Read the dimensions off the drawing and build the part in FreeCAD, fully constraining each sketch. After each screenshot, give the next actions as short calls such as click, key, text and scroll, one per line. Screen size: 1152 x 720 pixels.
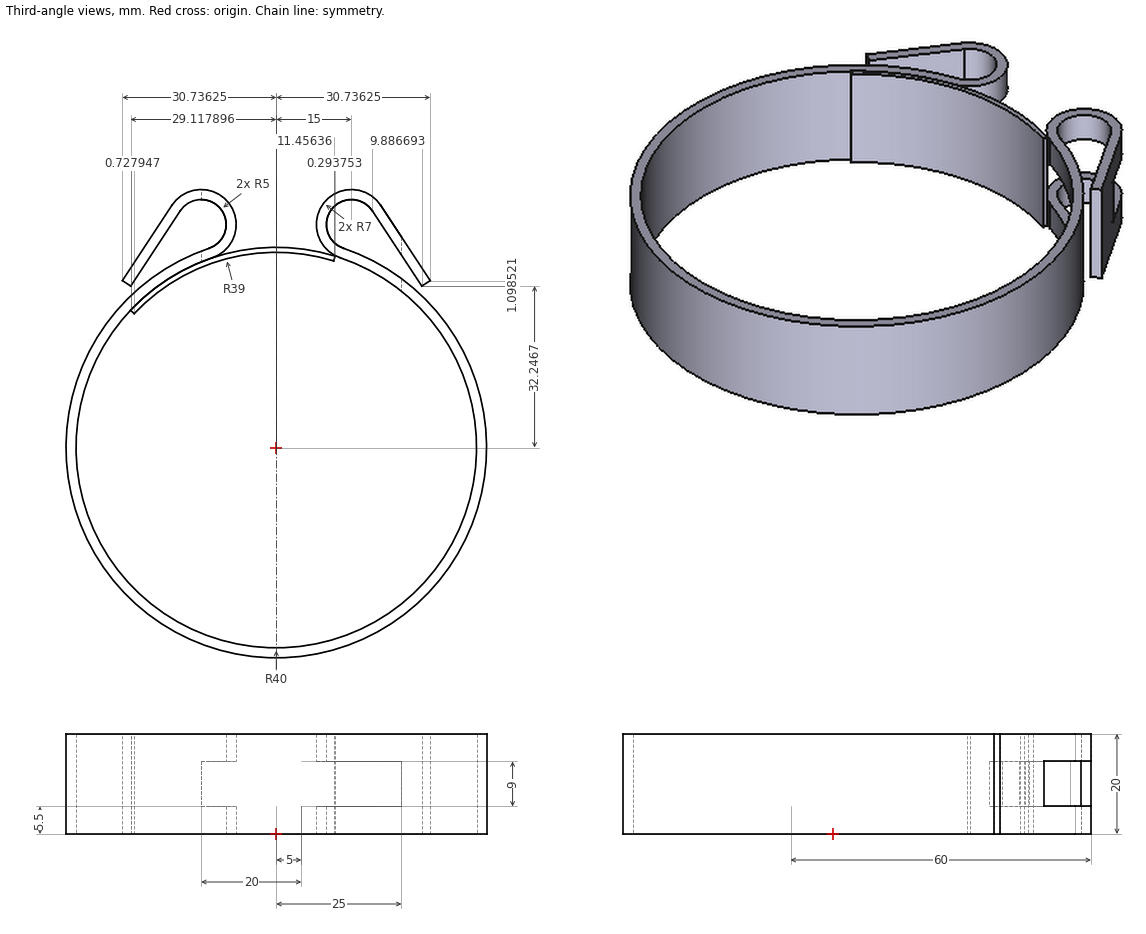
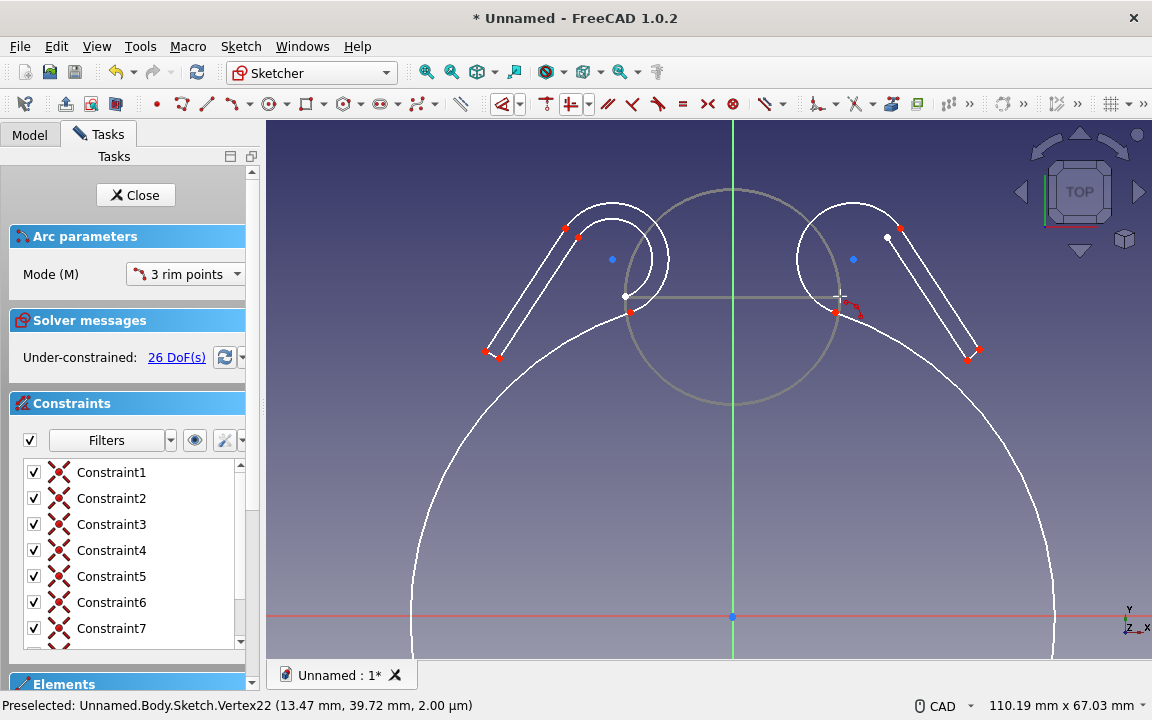
scroll(565, 227, down, 4)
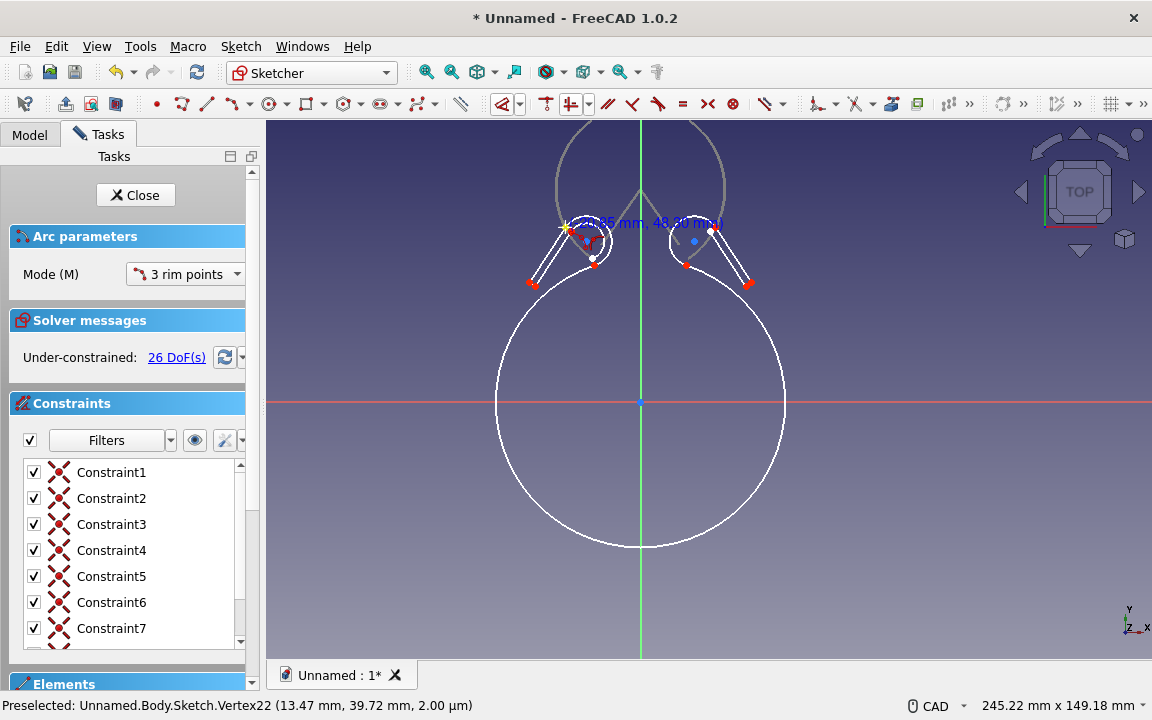
scroll(559, 530, up, 4)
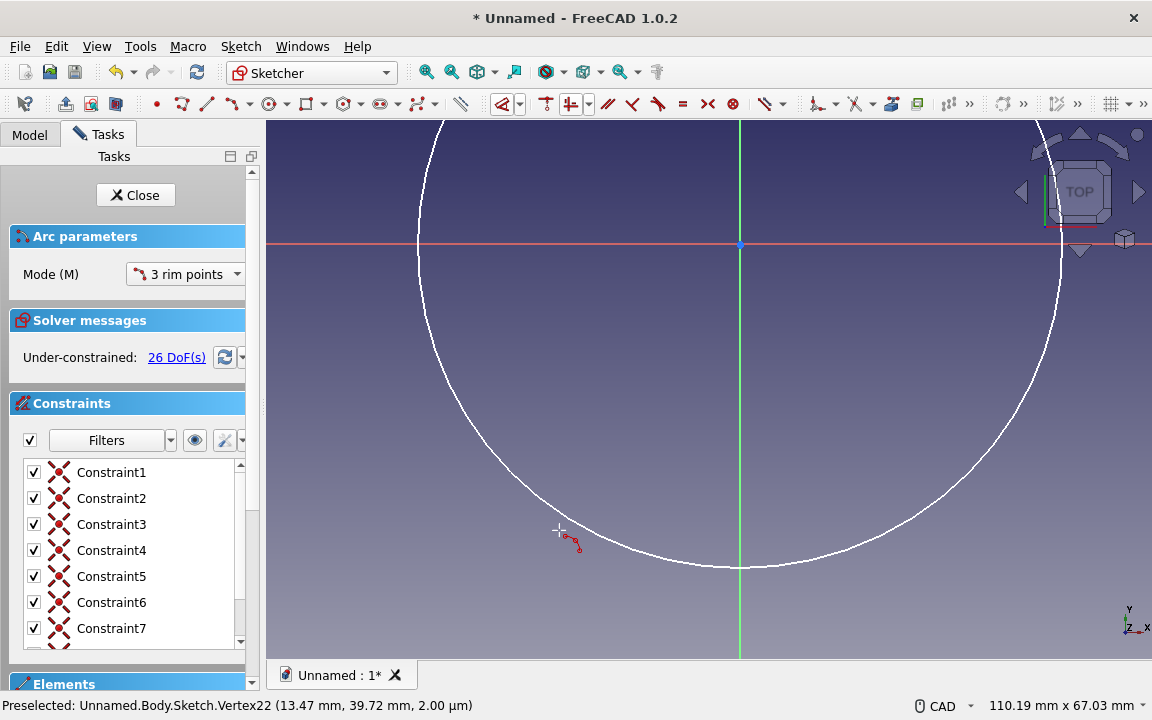
click(560, 530)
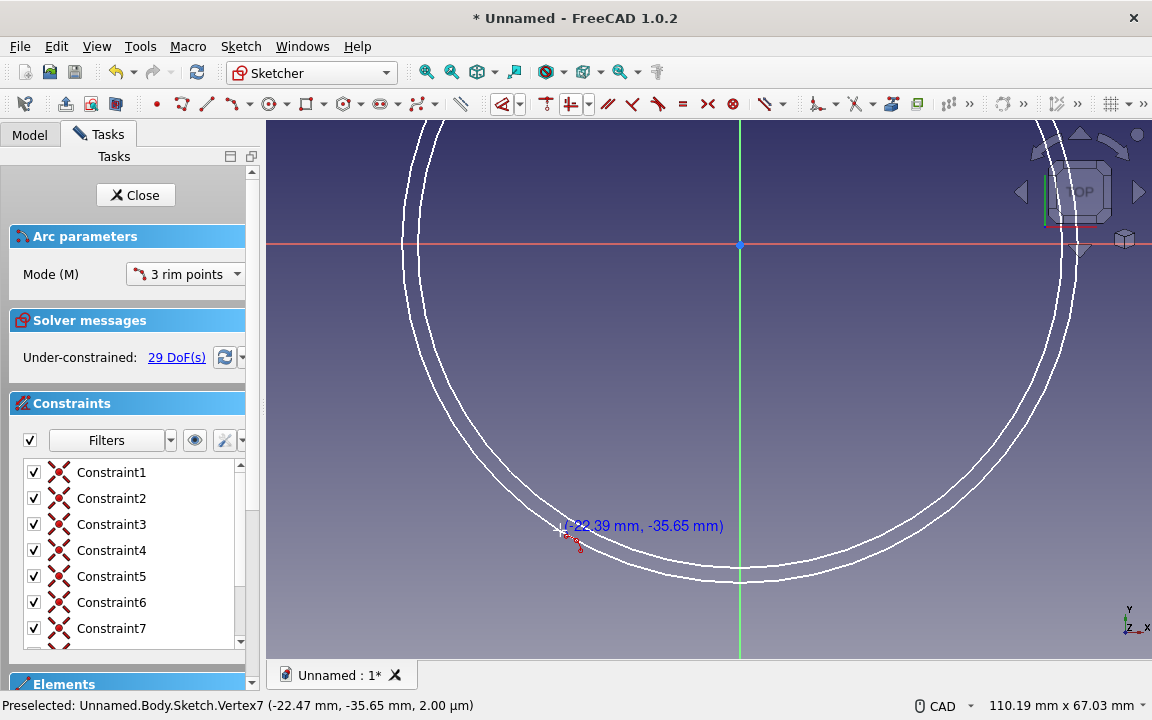
scroll(559, 530, down, 4)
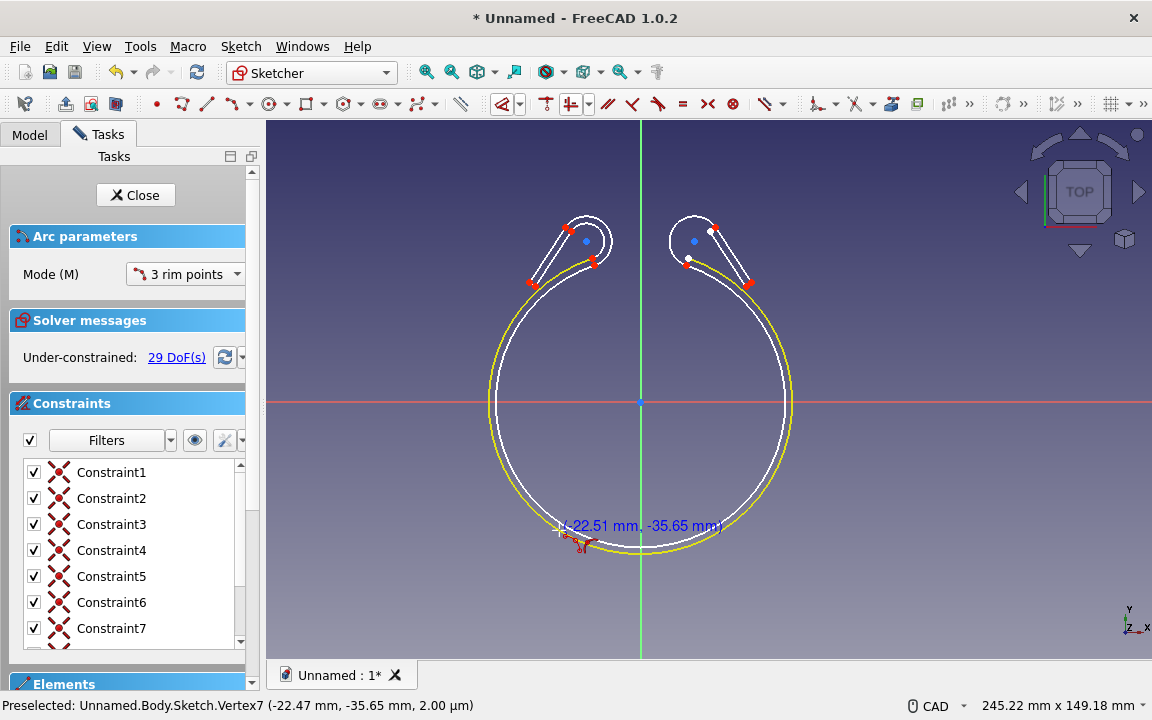
scroll(689, 258, up, 4)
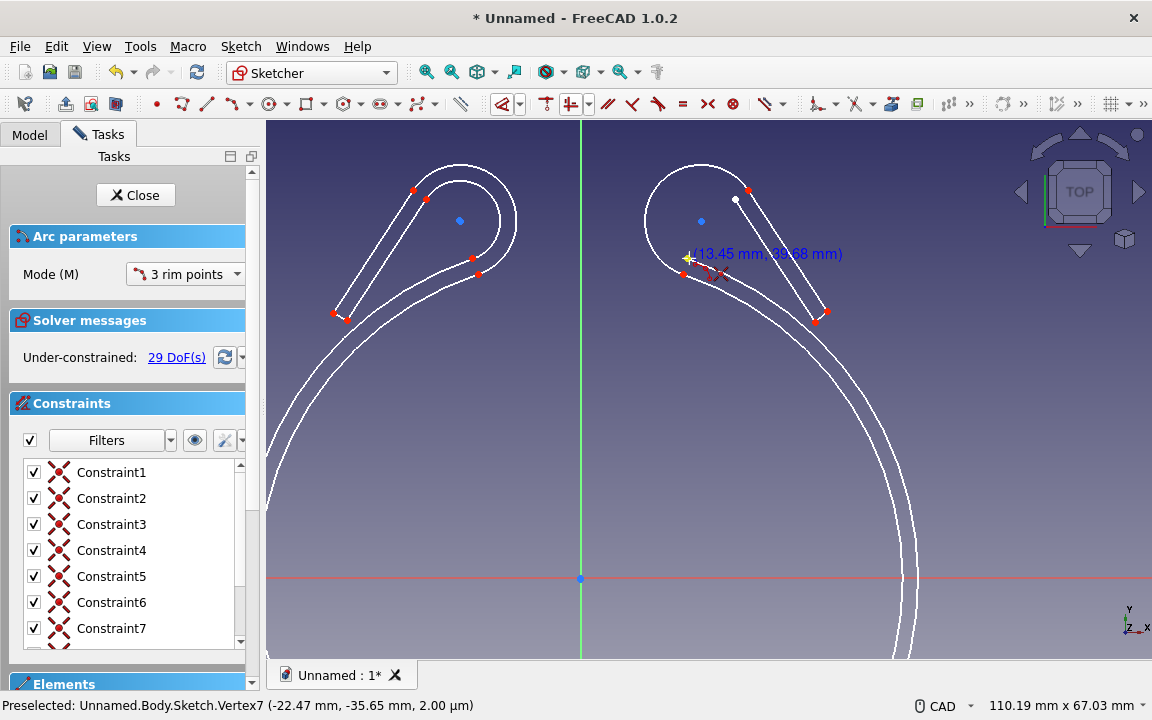
click(688, 259)
click(735, 200)
click(695, 180)
key(Escape)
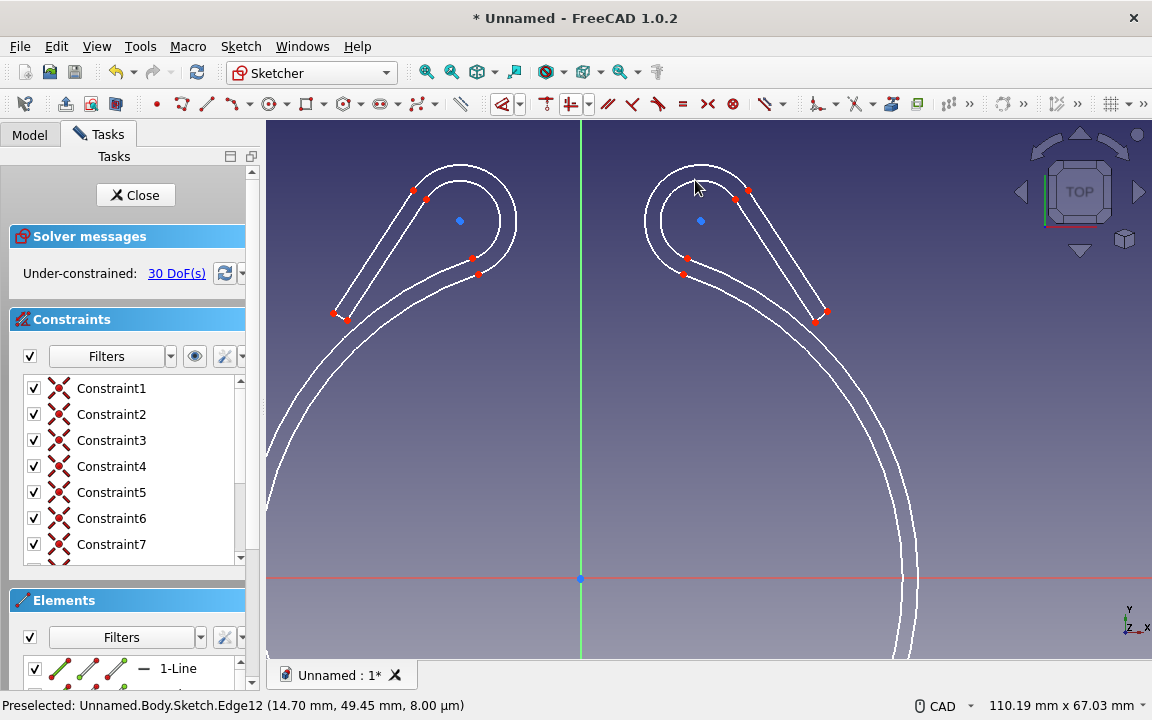
click(759, 237)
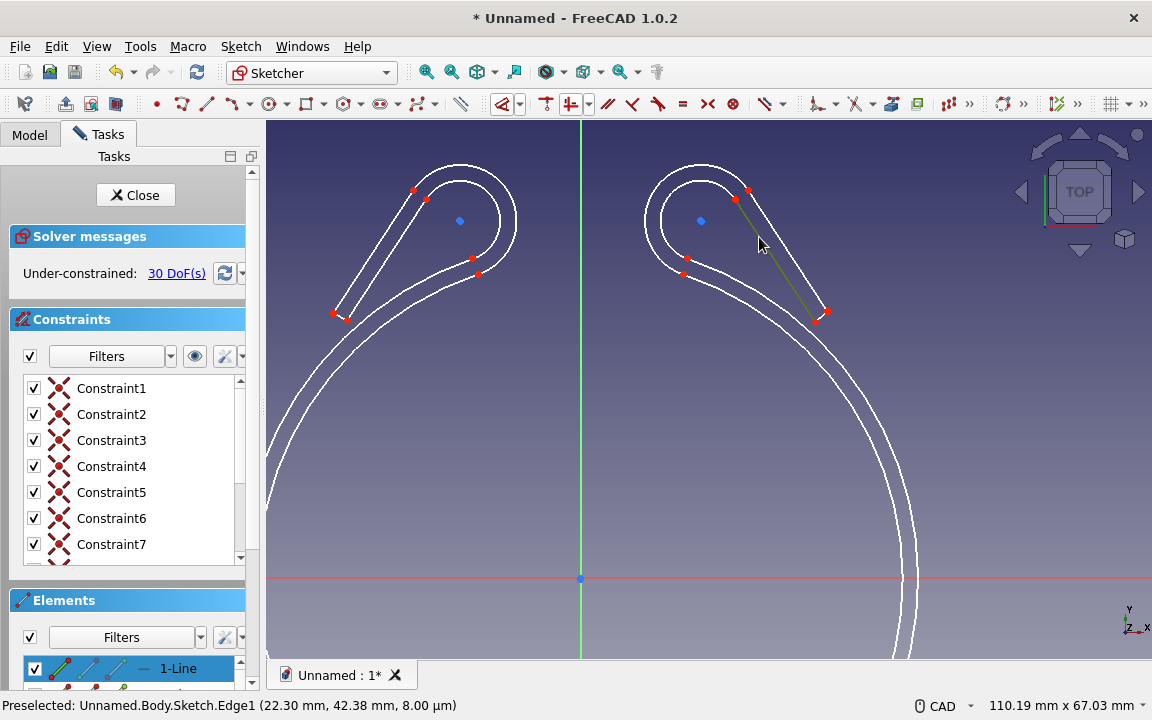
click(696, 181)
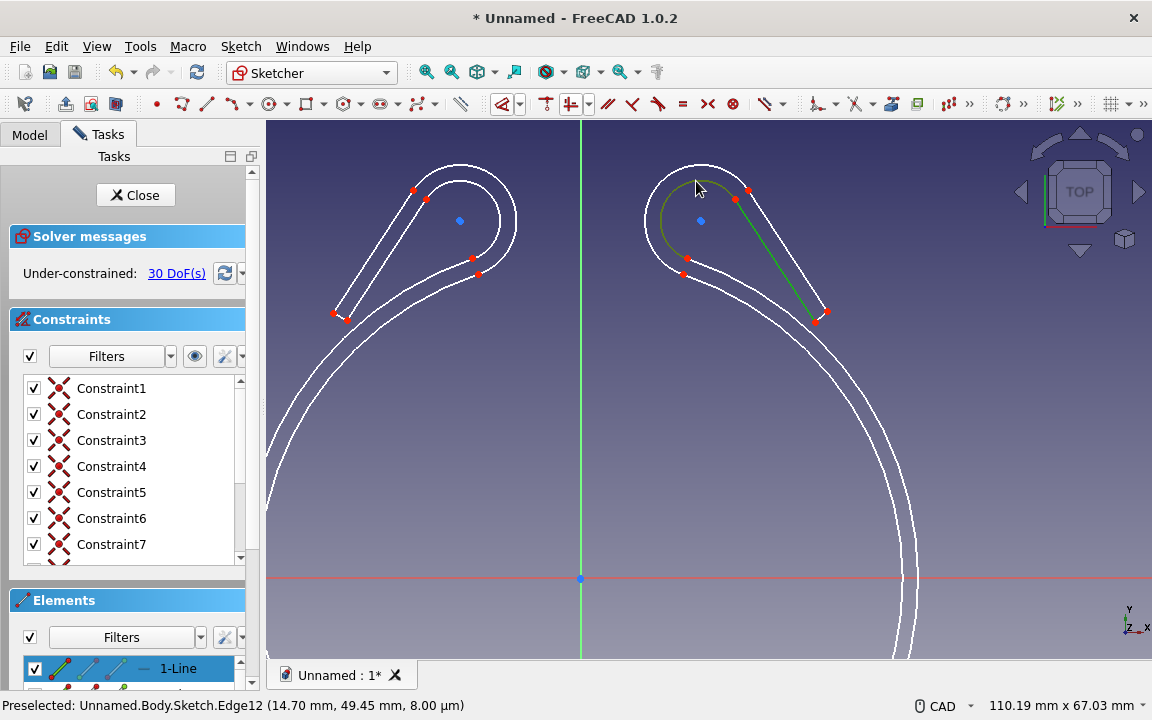
key(t)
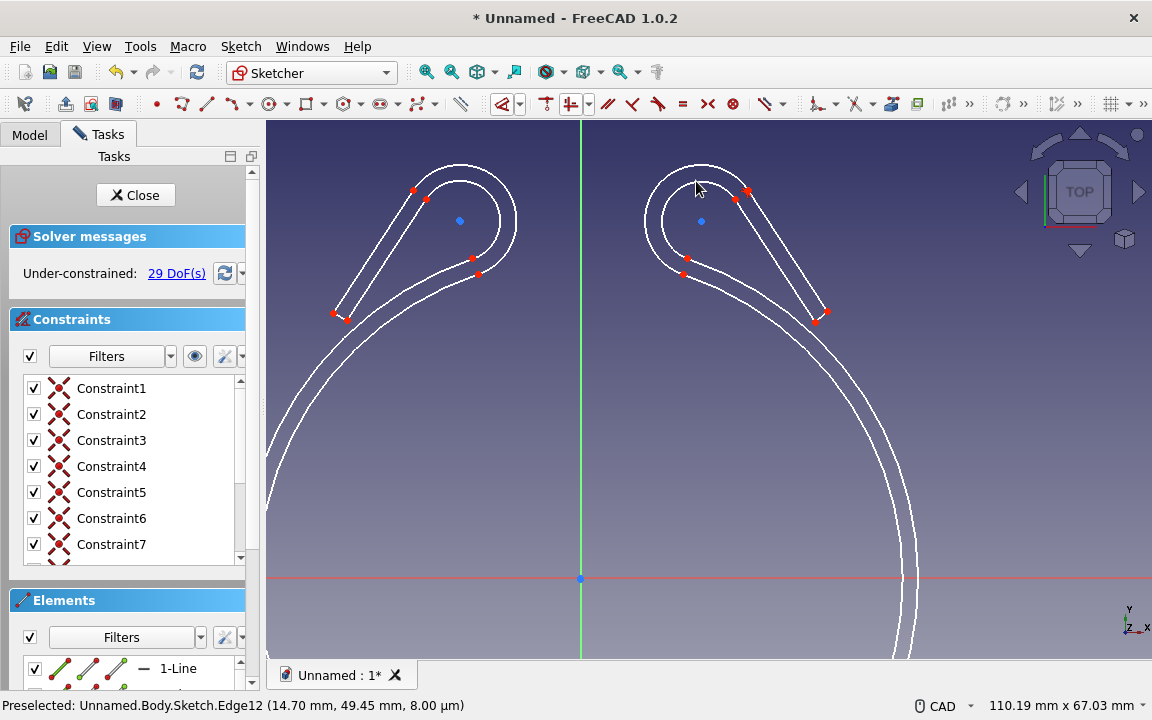
click(804, 275)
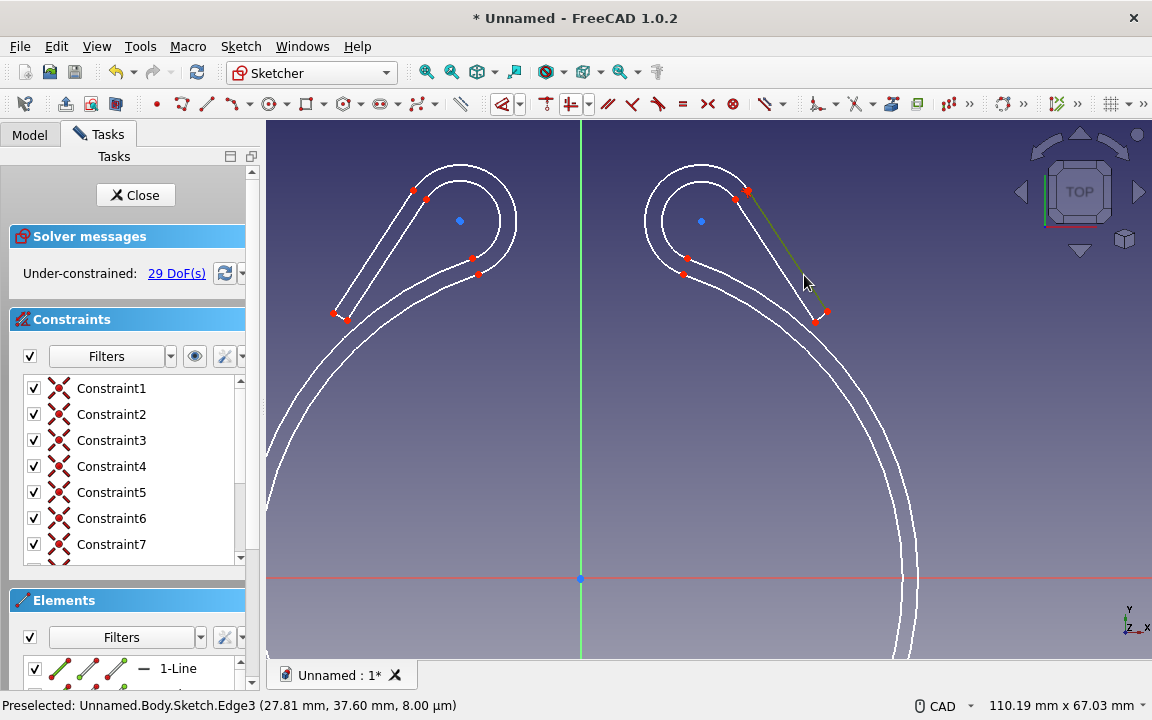
click(693, 166)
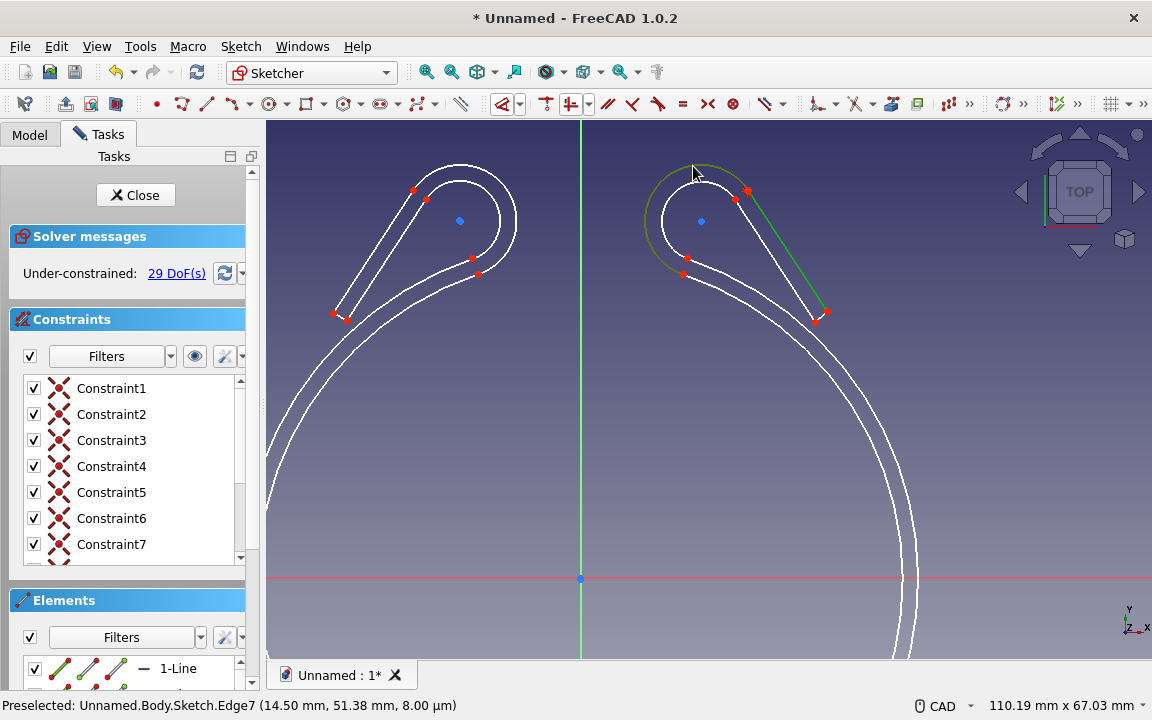
key(t)